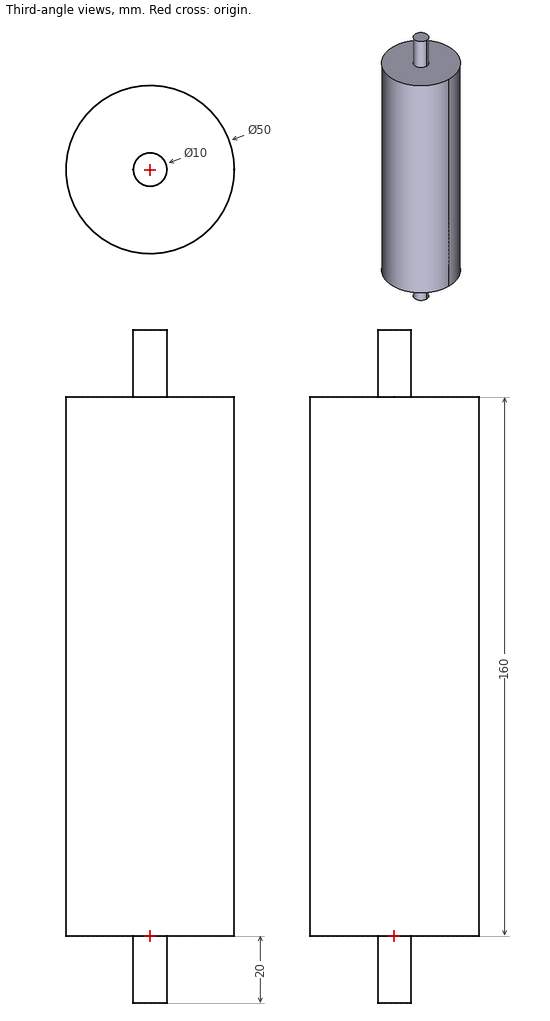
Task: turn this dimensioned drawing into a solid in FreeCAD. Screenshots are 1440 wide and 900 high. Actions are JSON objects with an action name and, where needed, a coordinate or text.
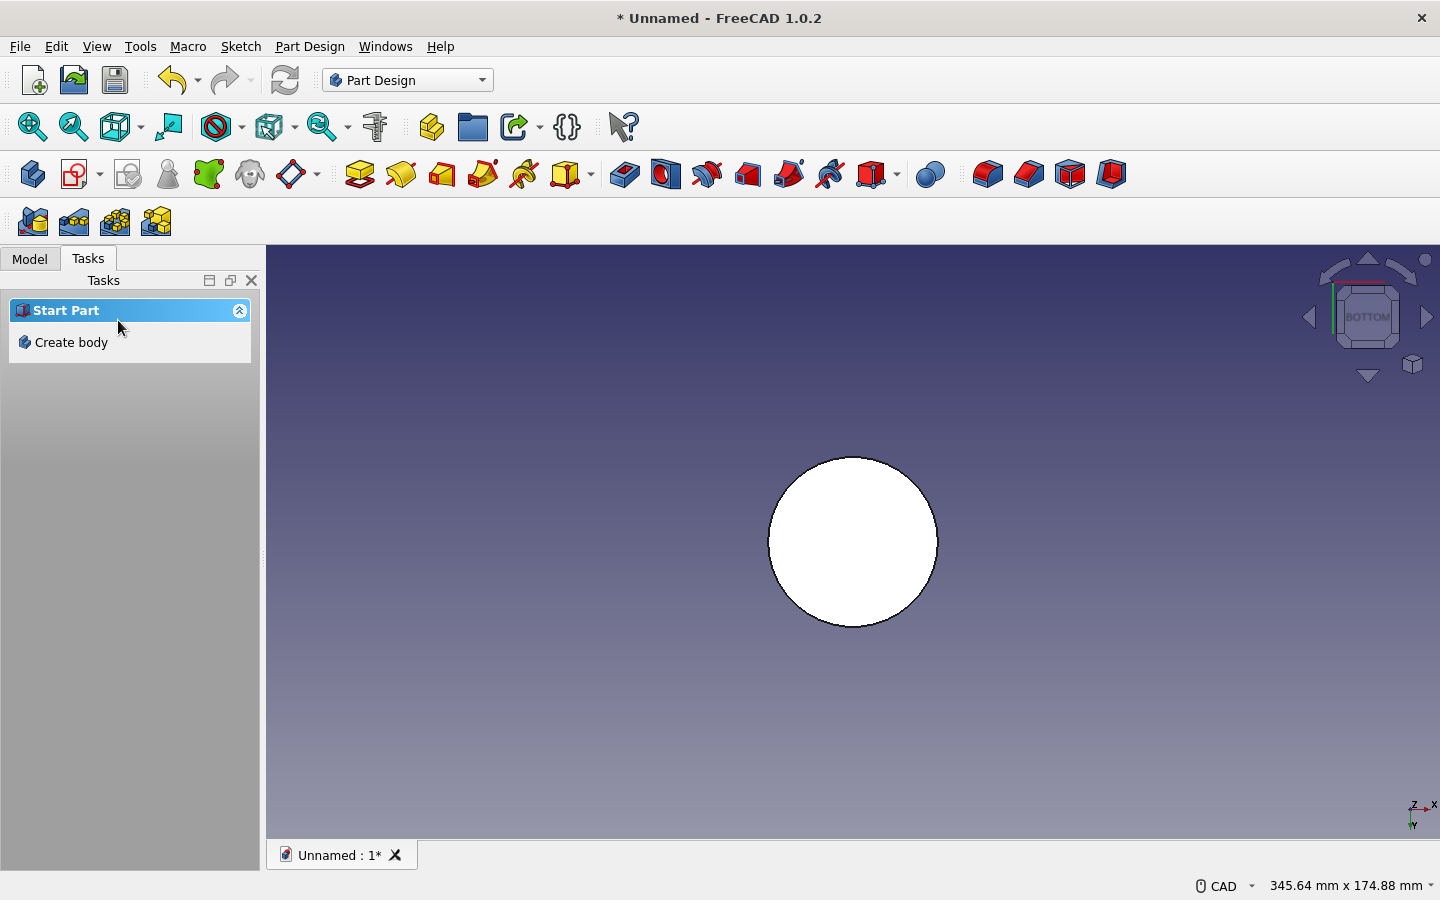
{"action": "left_click", "coordinate": [853, 541]}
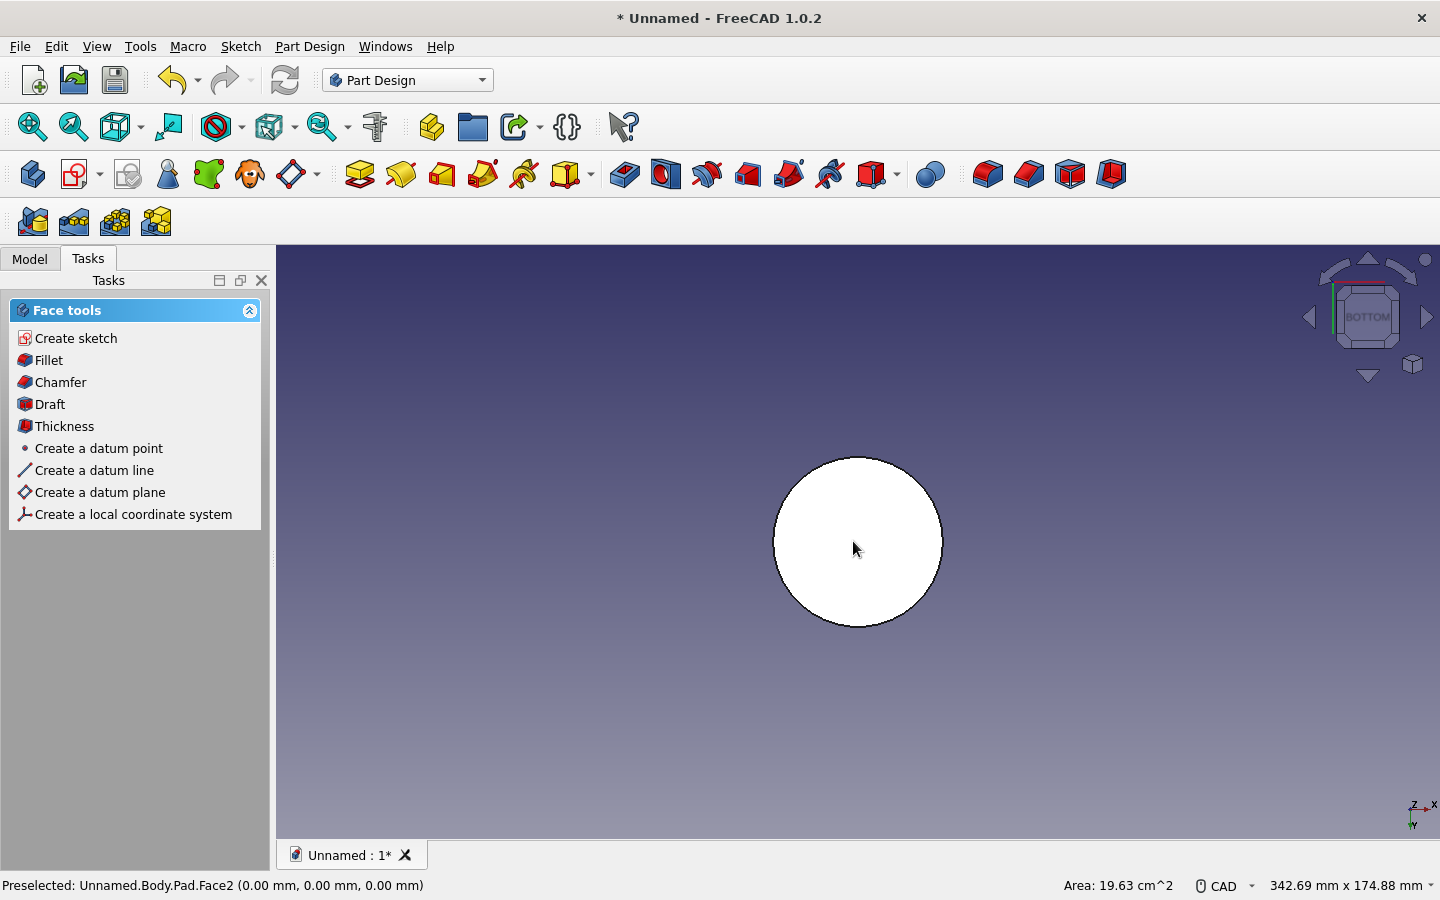
{"action": "left_click", "coordinate": [74, 174]}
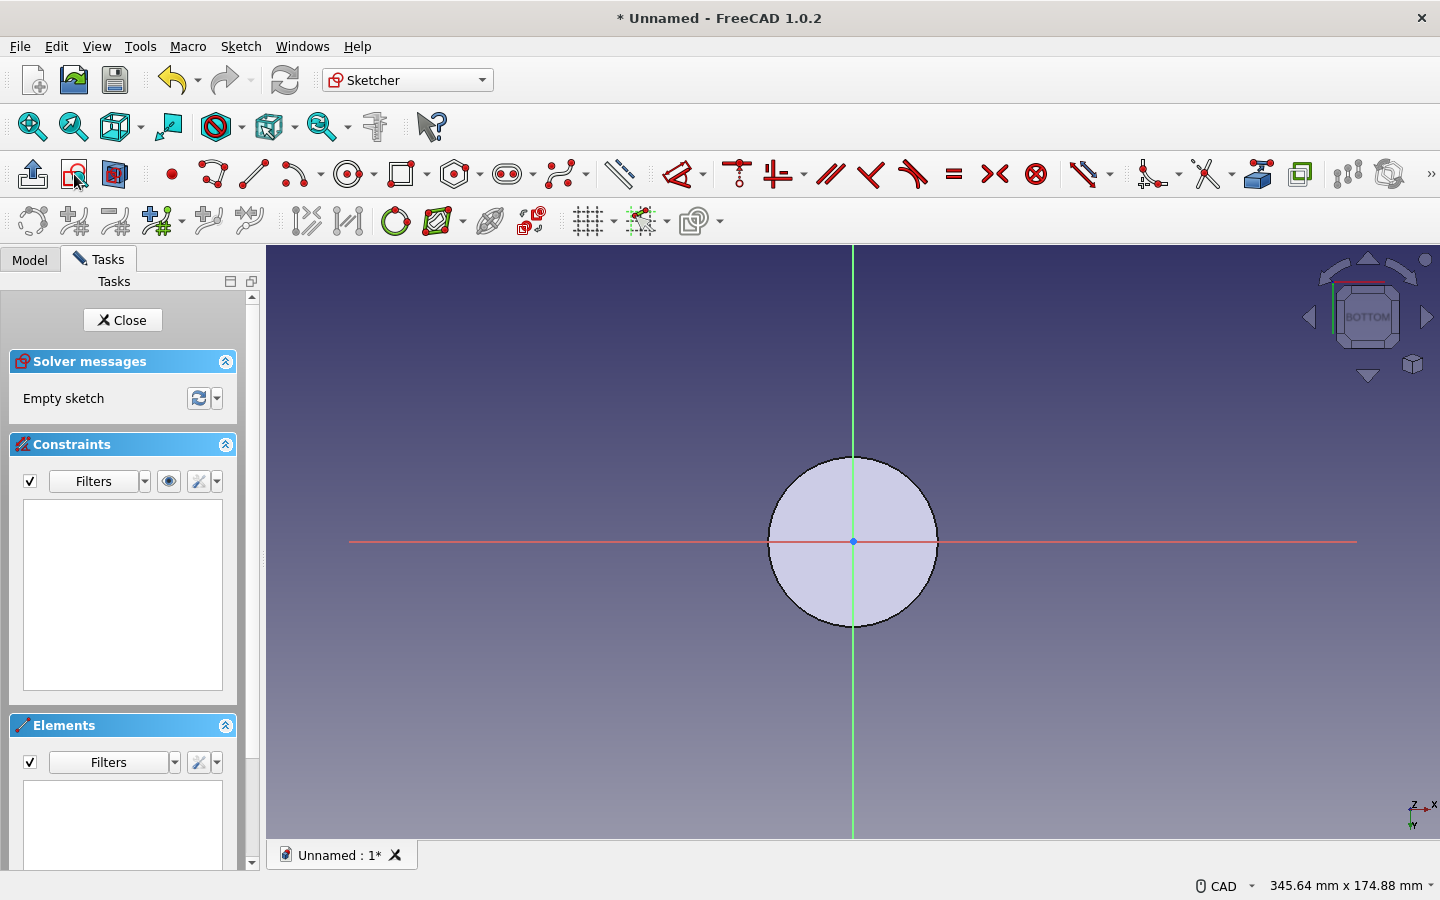
{"action": "scroll", "coordinate": [860, 542], "scroll_direction": "up", "scroll_amount": 12}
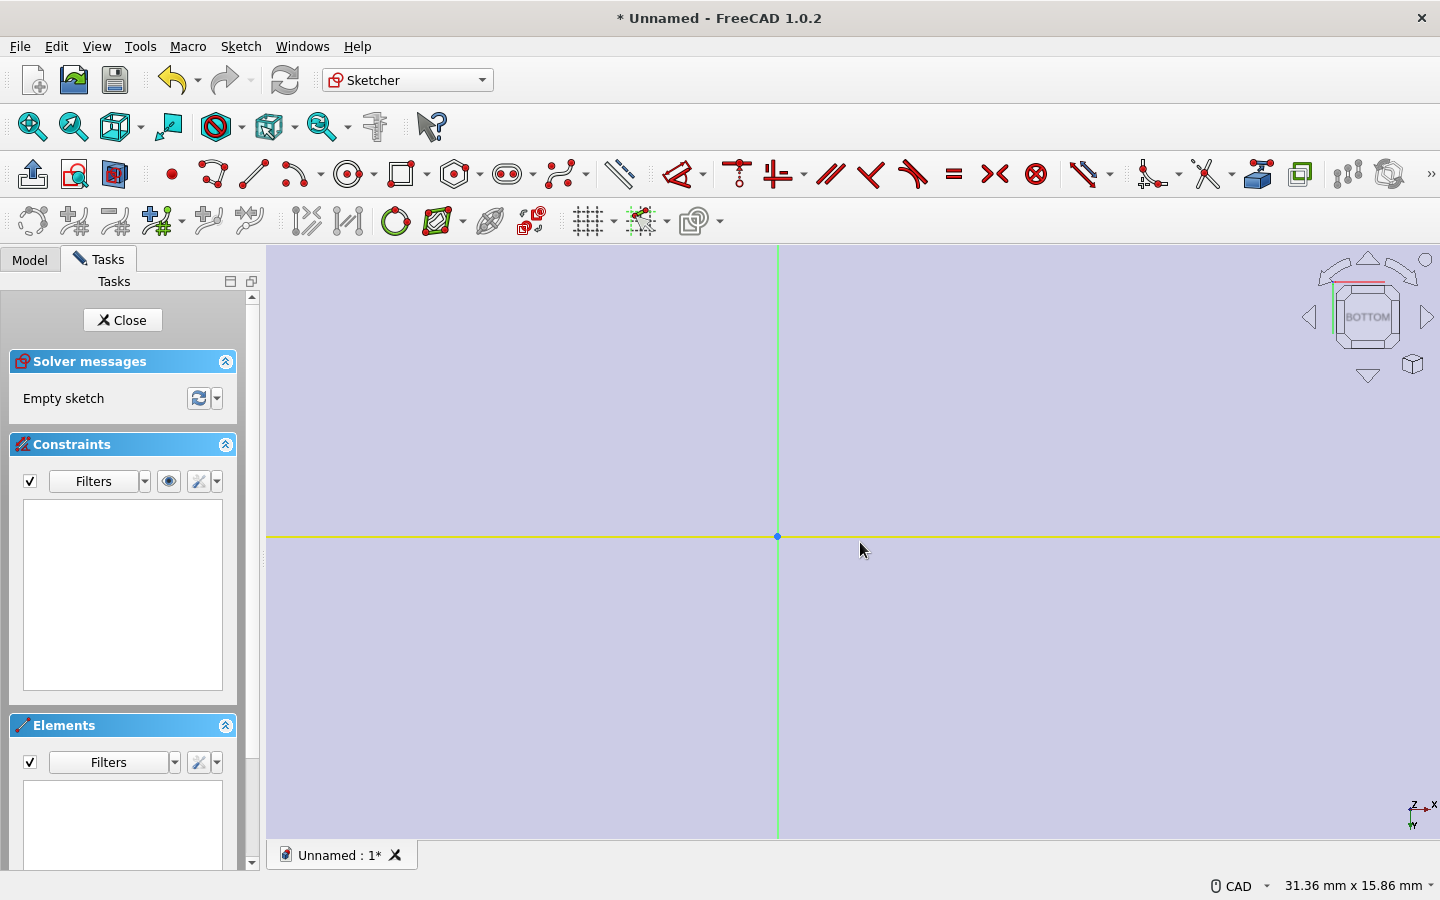
{"action": "key", "text": "g c"}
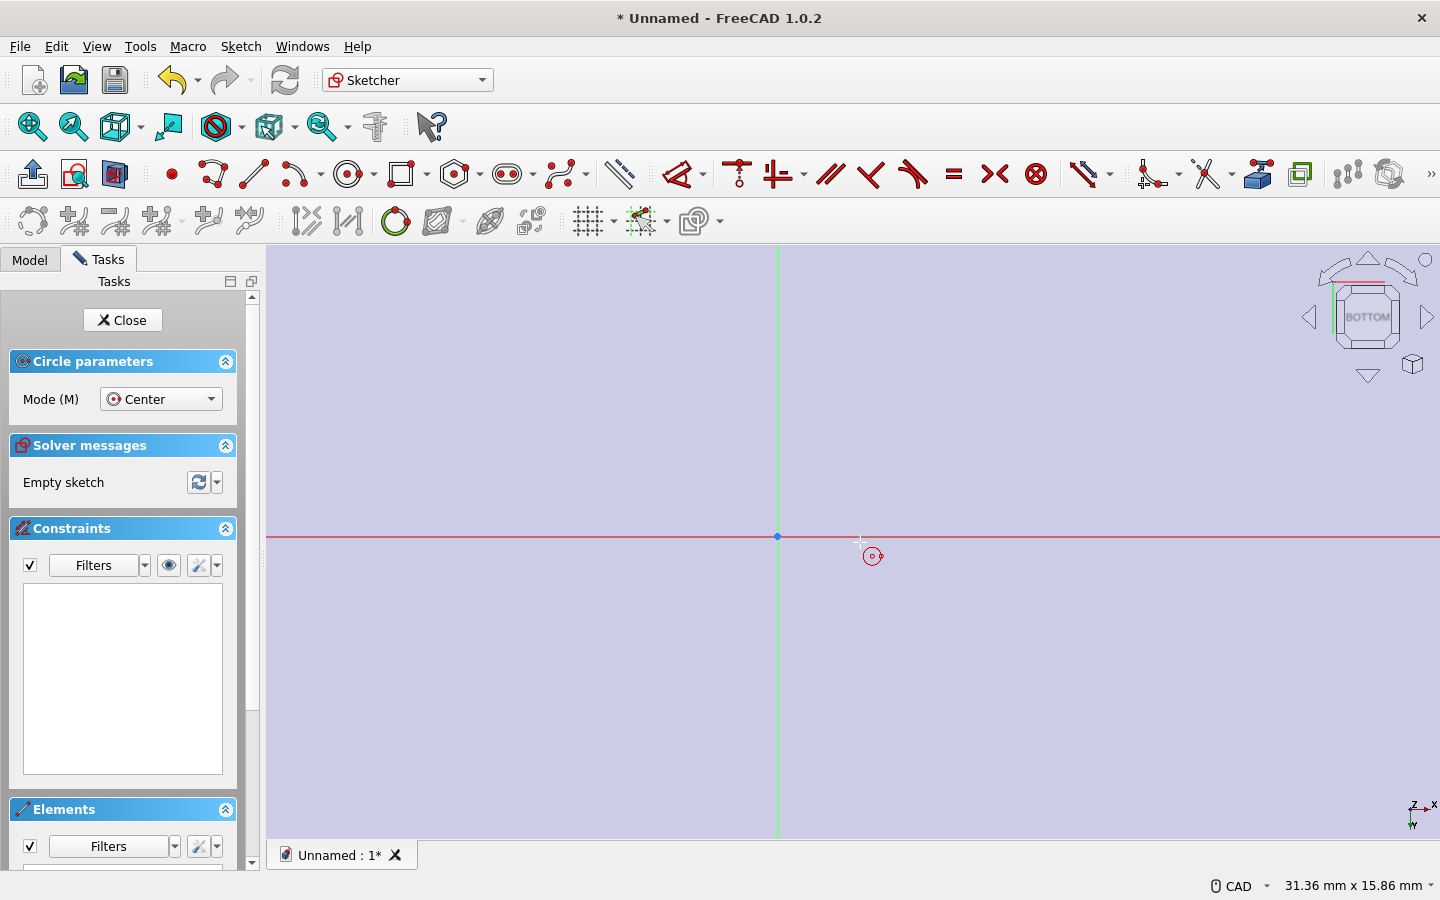
{"action": "left_click", "coordinate": [778, 537]}
{"action": "left_click", "coordinate": [910, 405]}
{"action": "key", "text": "Escape"}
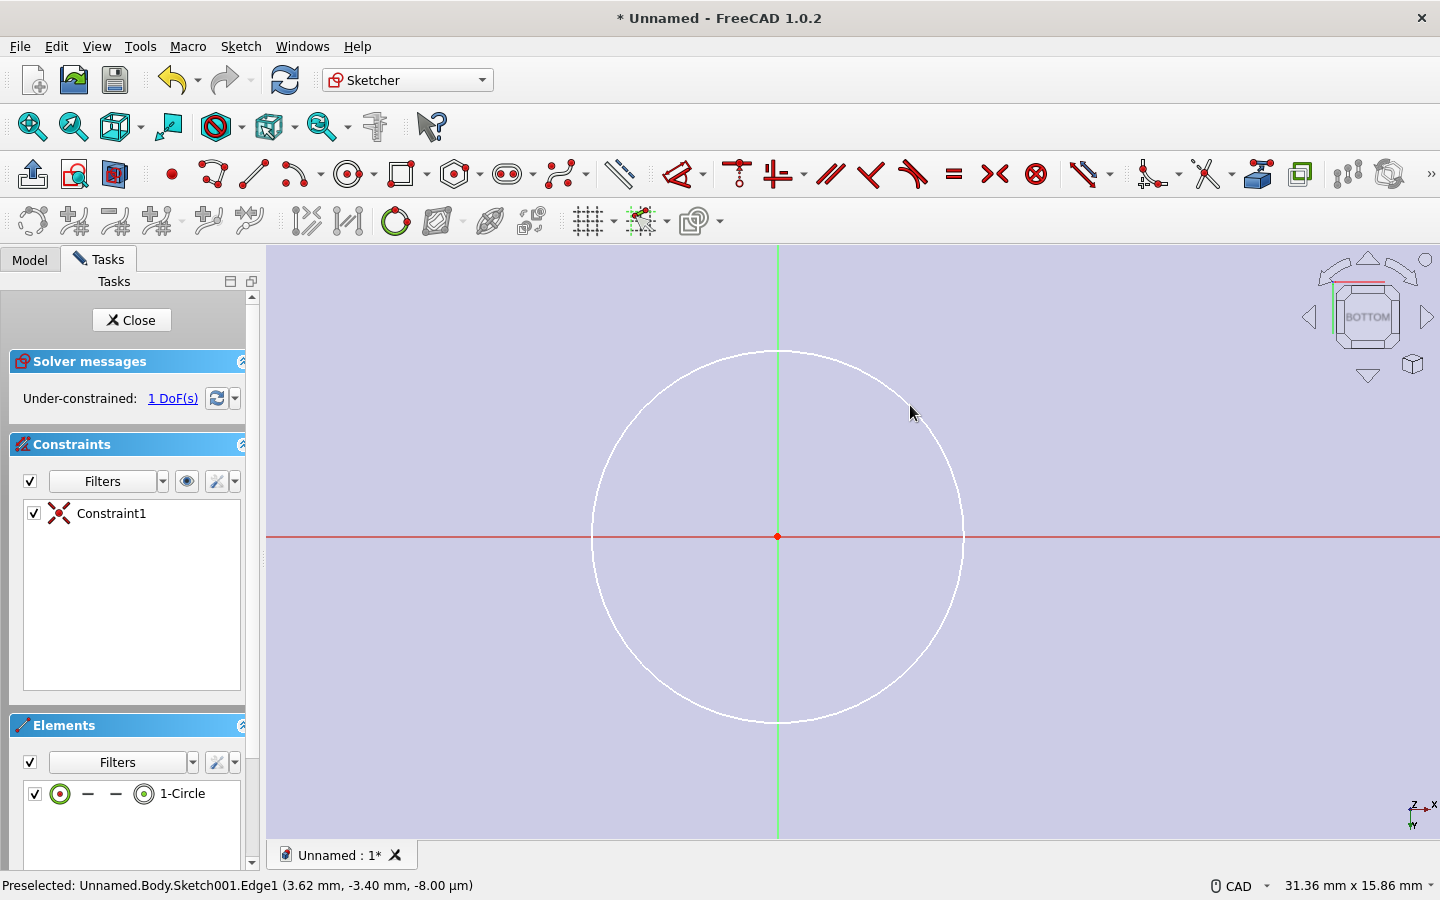
{"action": "key", "text": "d"}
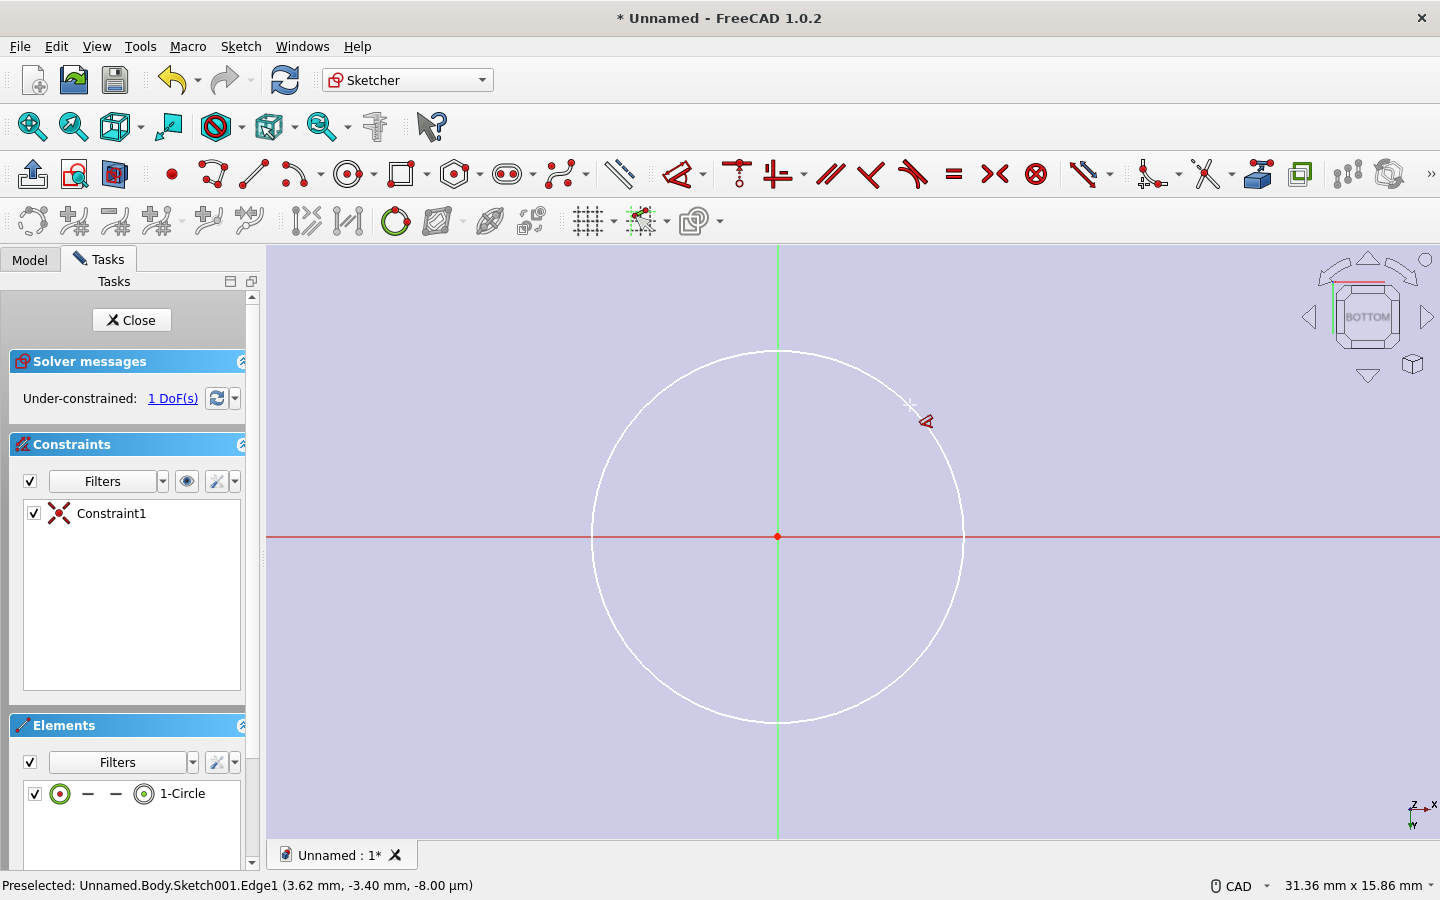
{"action": "left_click", "coordinate": [909, 405]}
{"action": "left_click", "coordinate": [932, 382]}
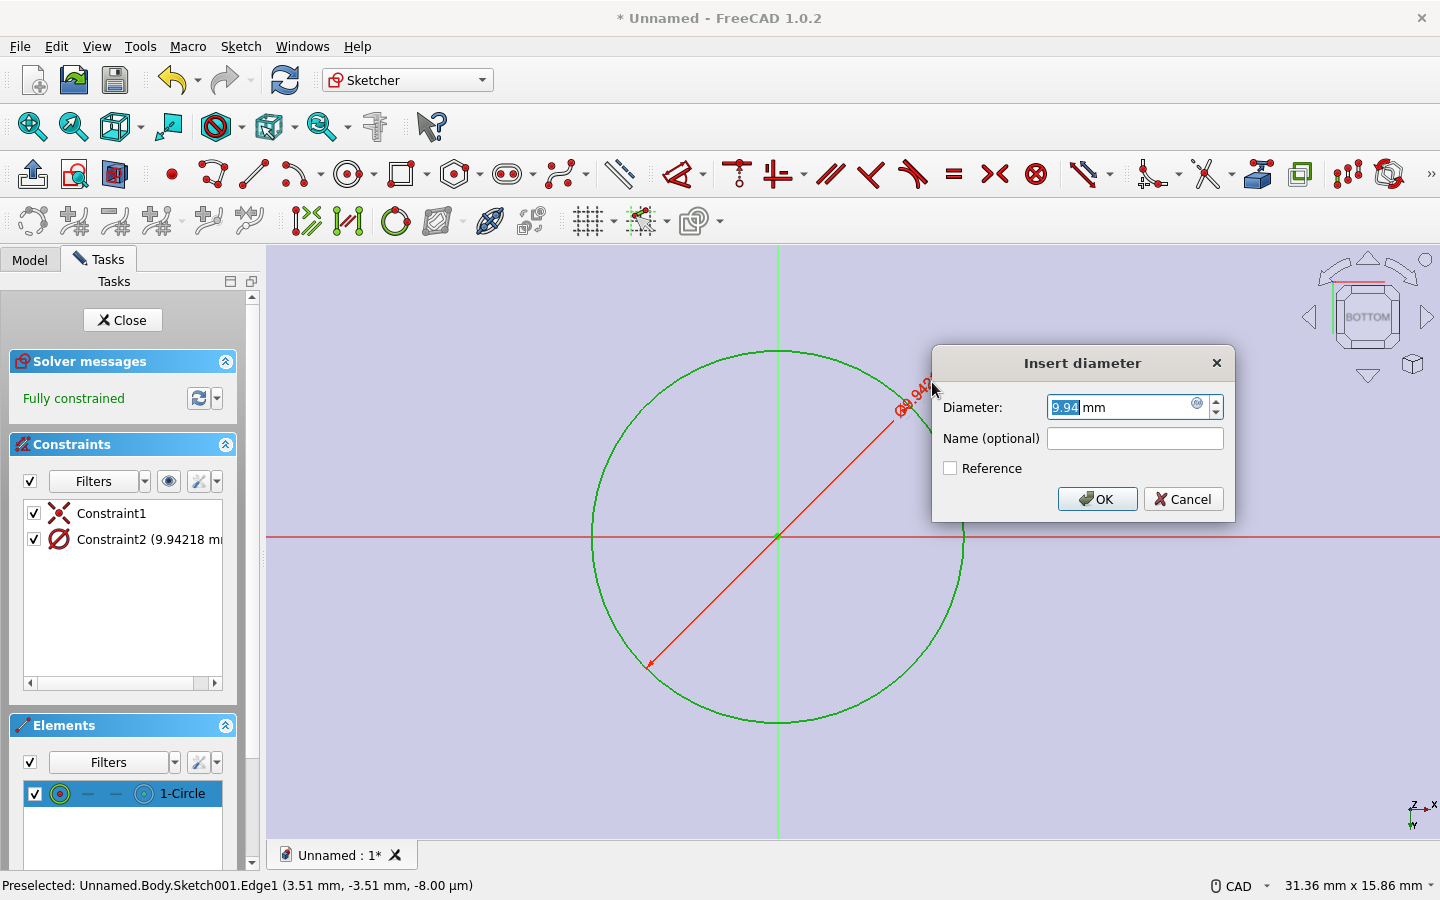
{"action": "type", "text": "10"}
{"action": "key", "text": "Return"}
{"action": "key", "text": "Escape"}